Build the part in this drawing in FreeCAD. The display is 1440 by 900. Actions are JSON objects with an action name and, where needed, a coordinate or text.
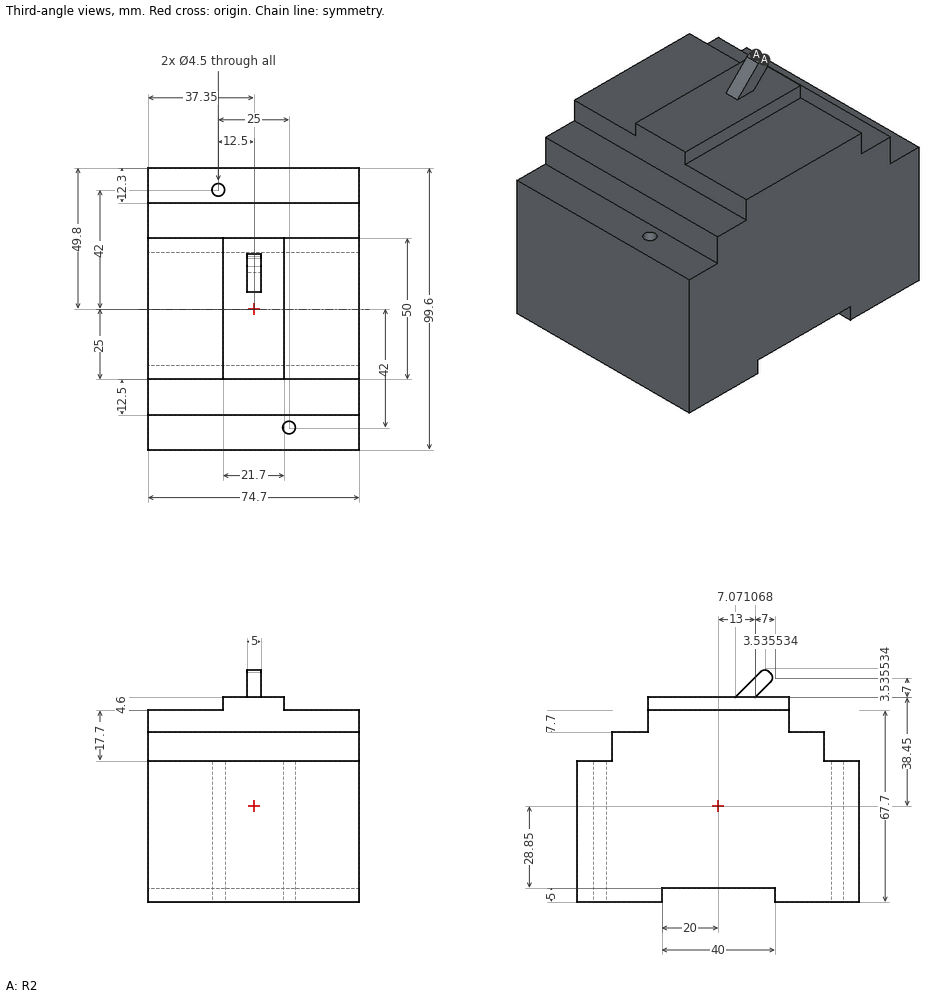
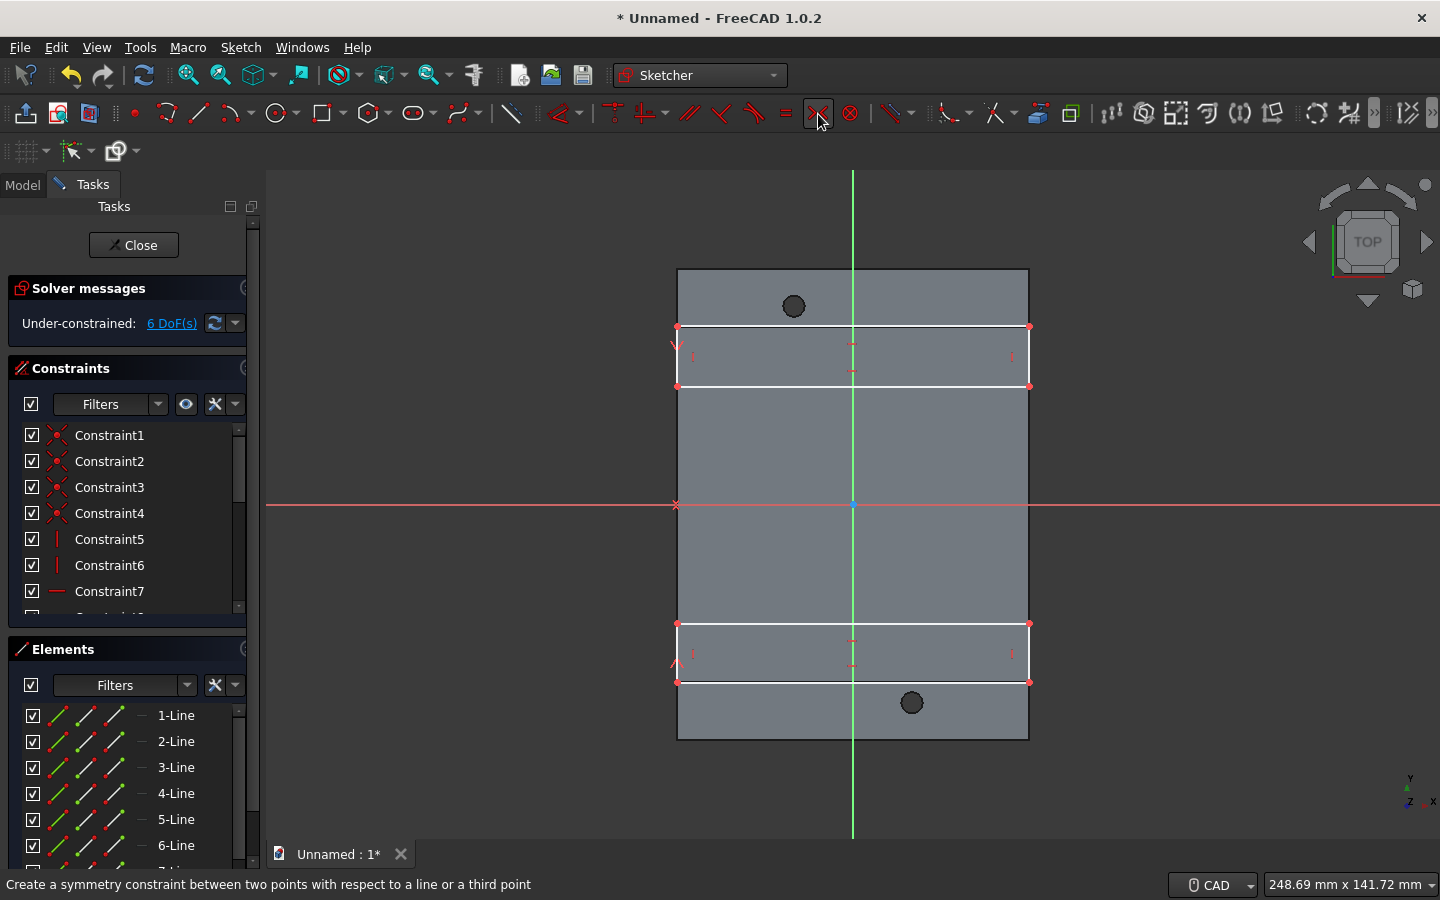
{"action": "left_click", "coordinate": [1029, 624]}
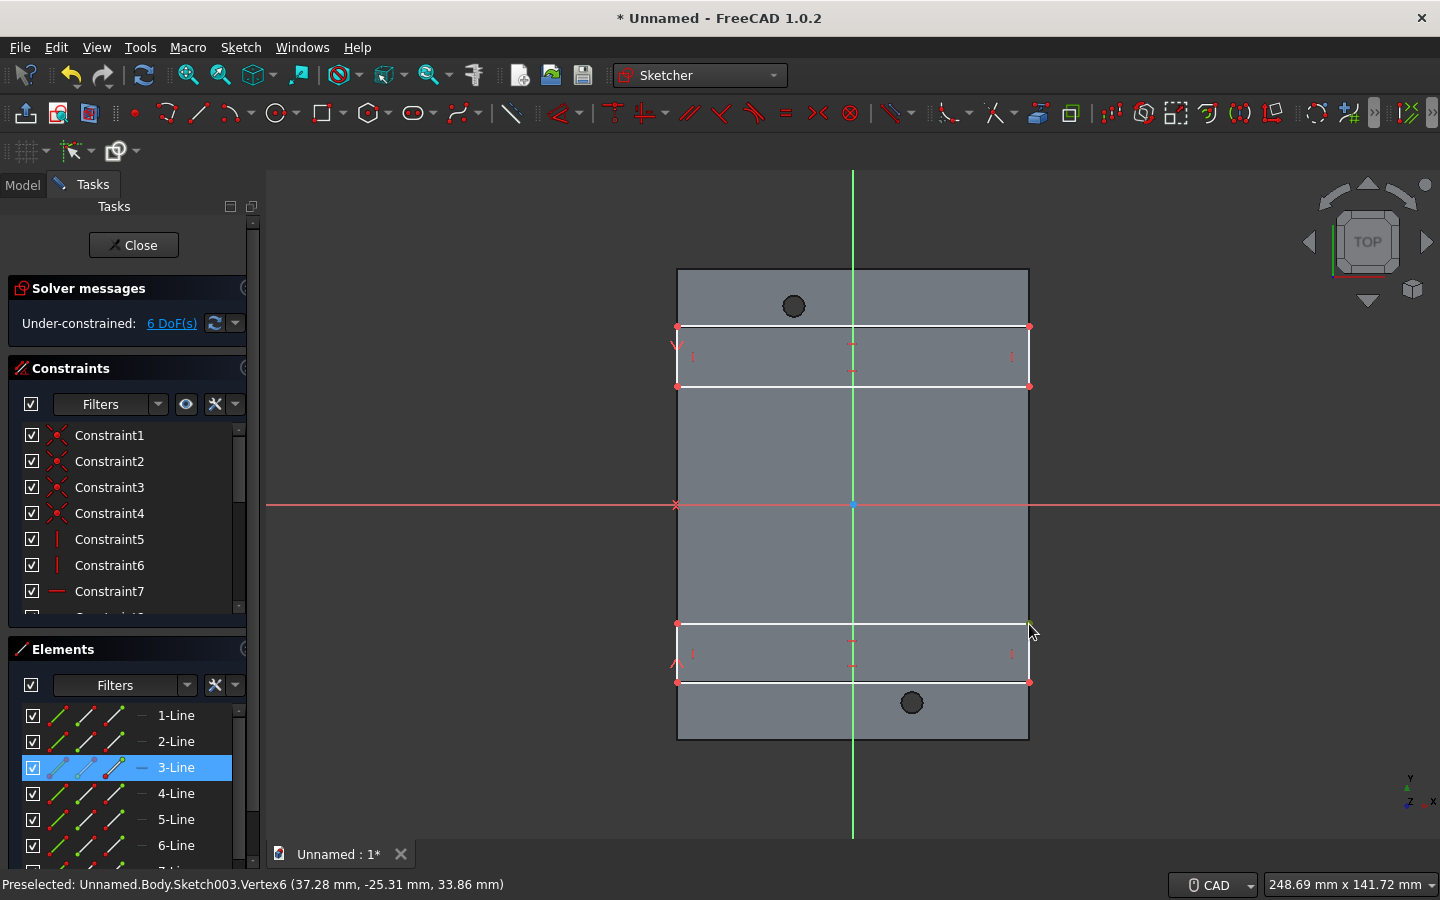
{"action": "left_click", "coordinate": [1029, 387]}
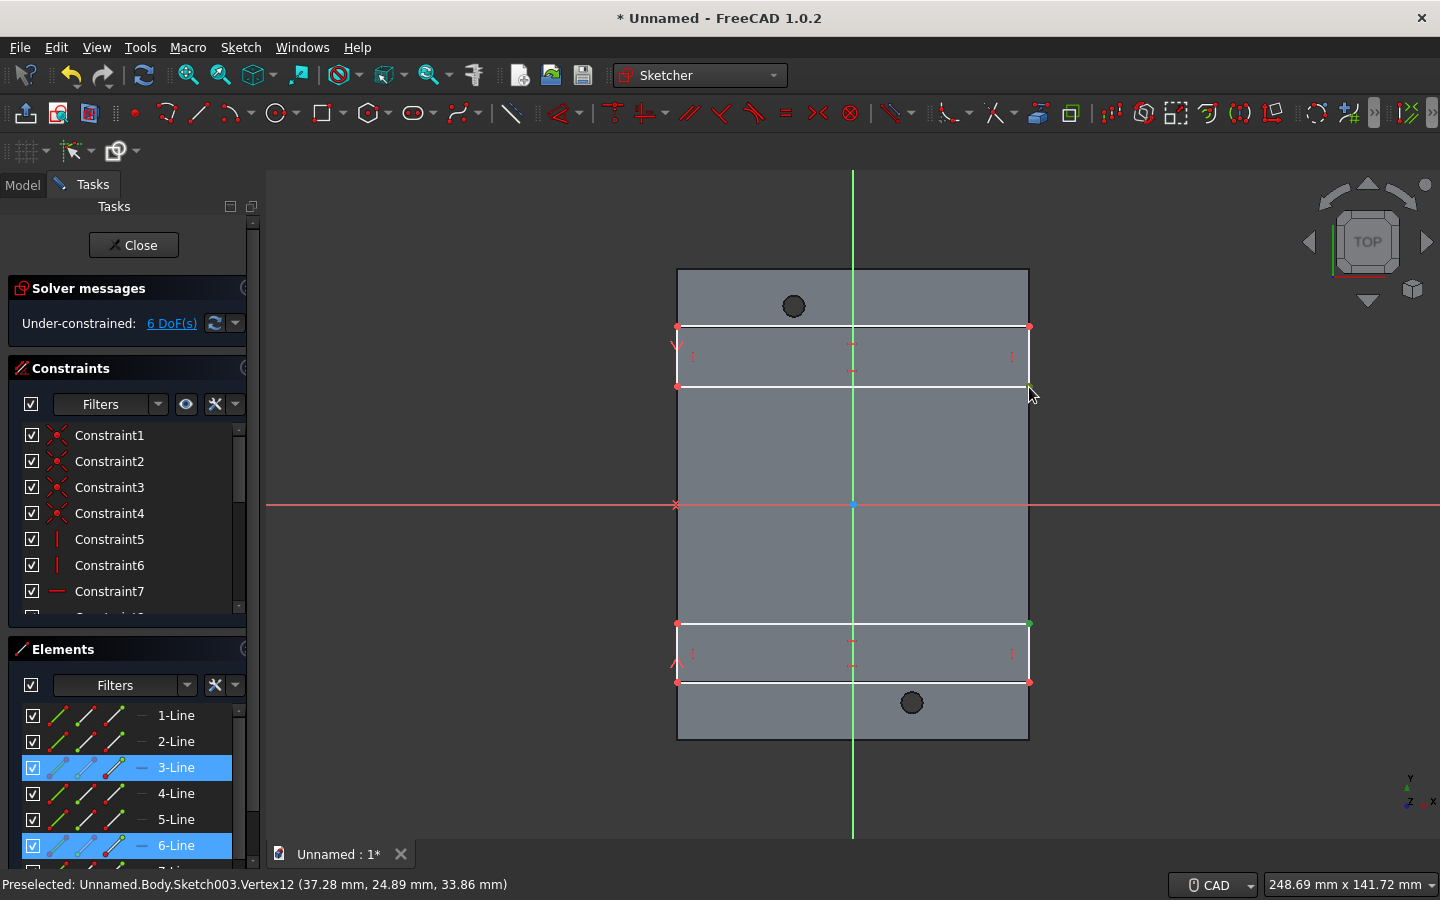
{"action": "left_click", "coordinate": [364, 504]}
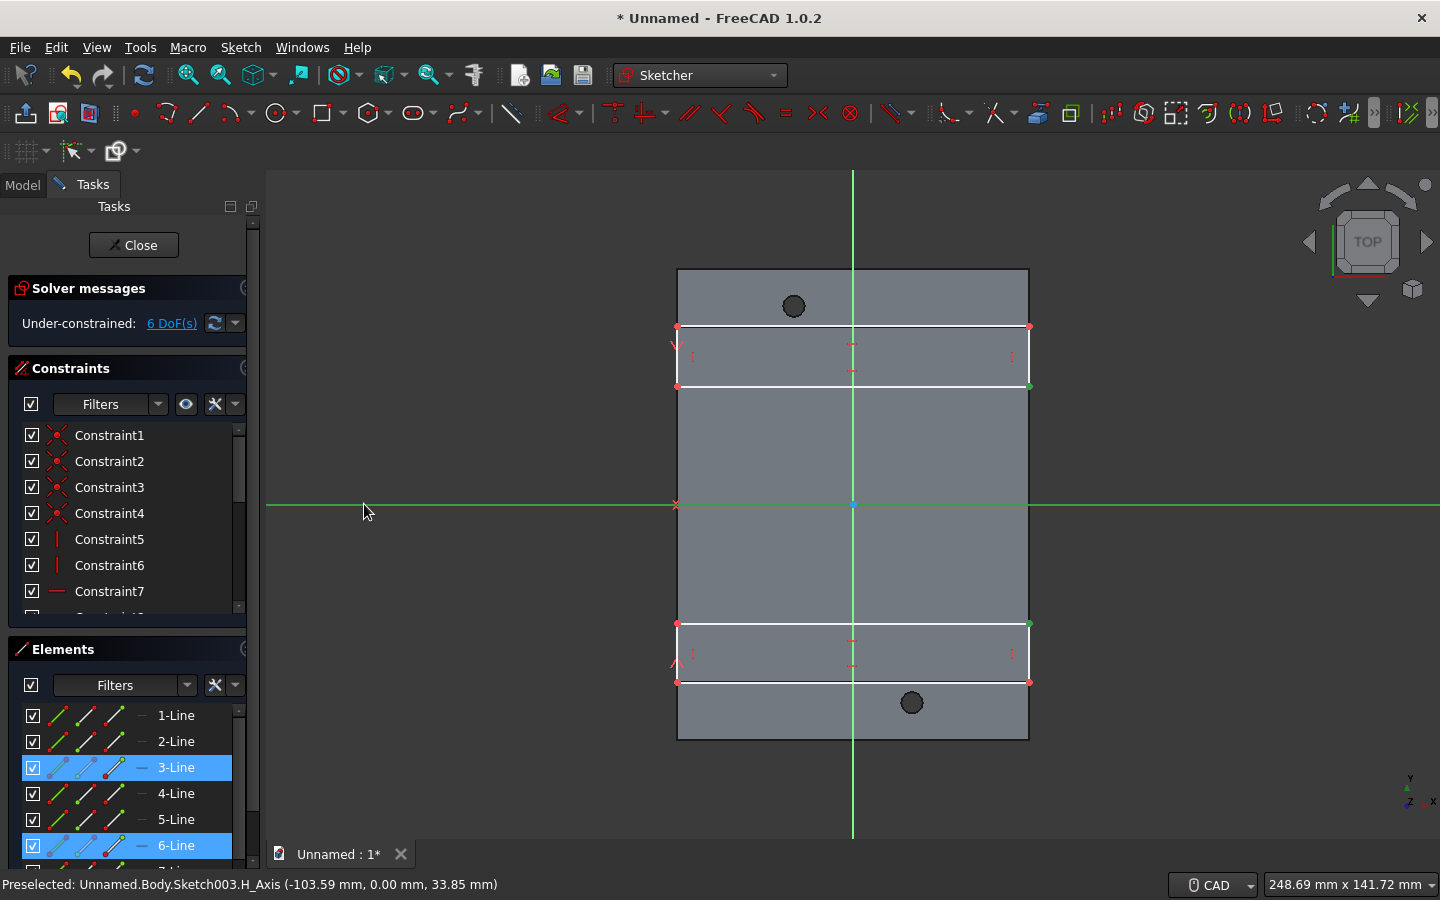
{"action": "left_click", "coordinate": [818, 114]}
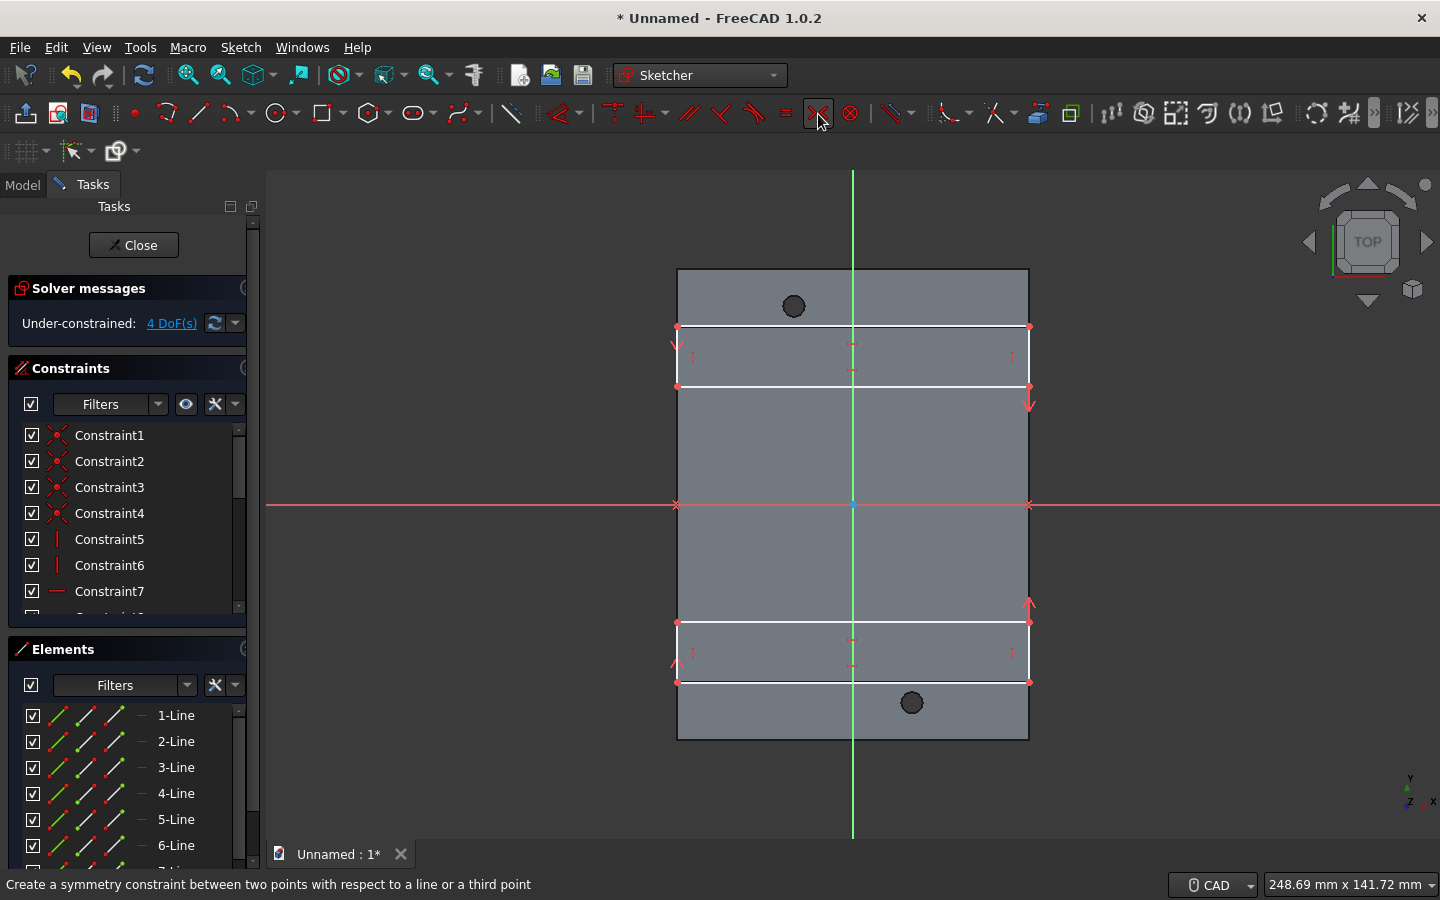
{"action": "left_click", "coordinate": [558, 114]}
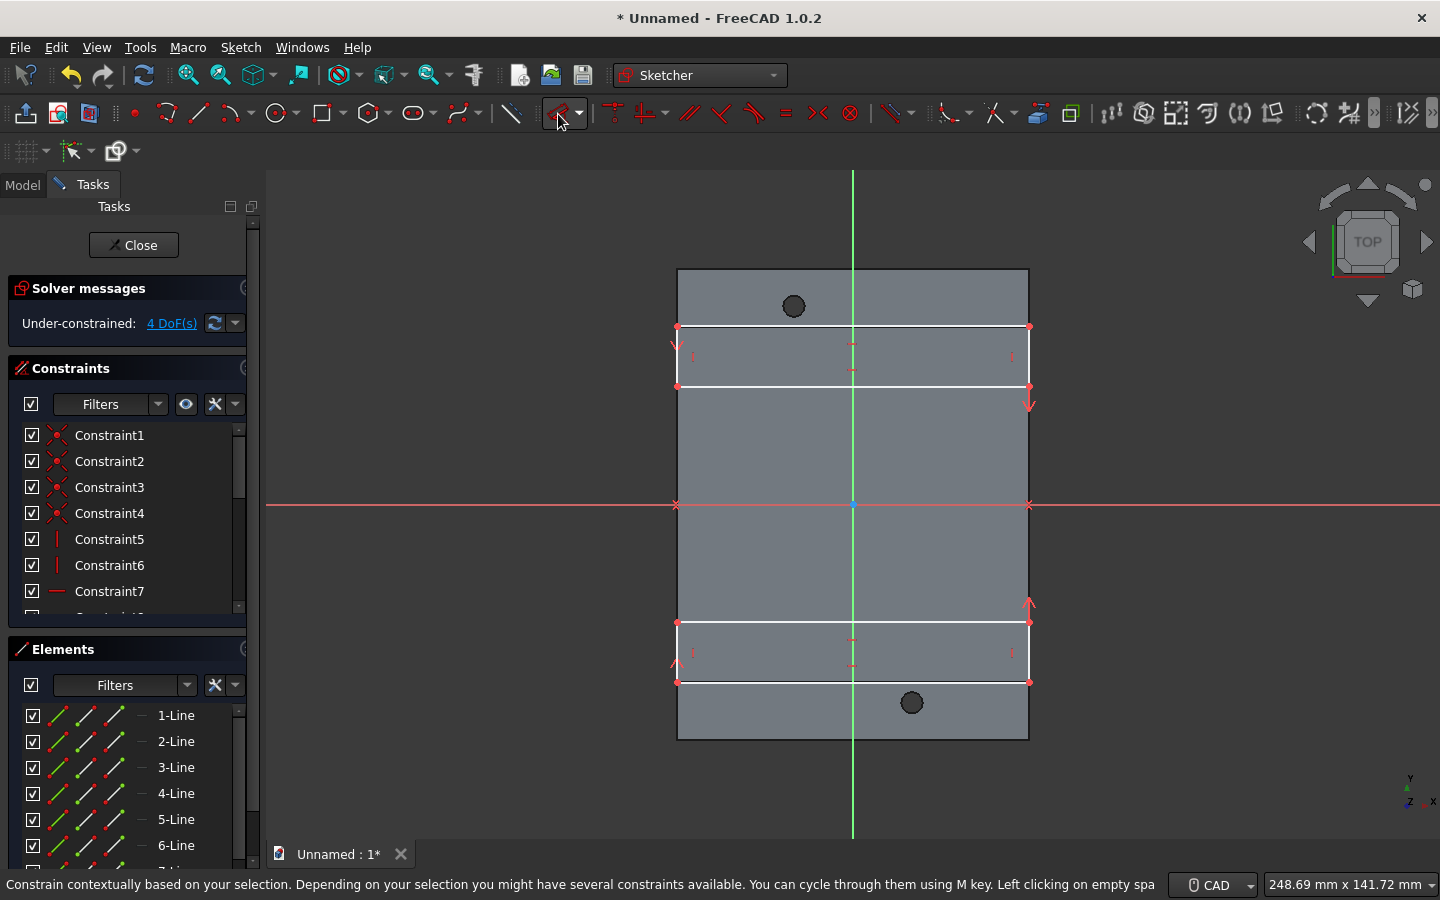
{"action": "left_click", "coordinate": [677, 622]}
{"action": "left_click", "coordinate": [643, 563]}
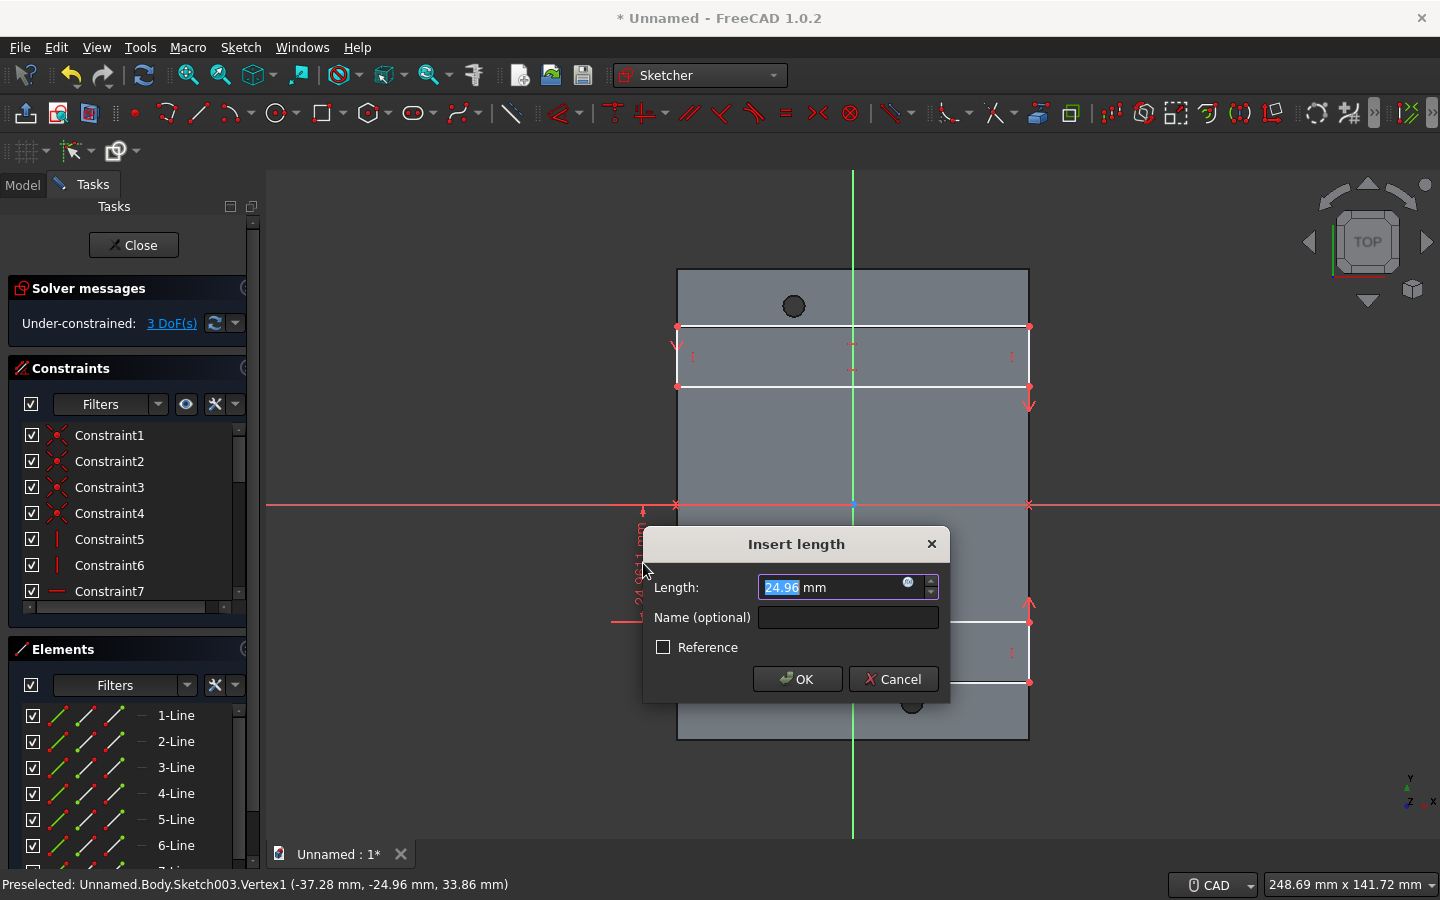
{"action": "type", "text": "25"}
{"action": "key", "text": "Return"}